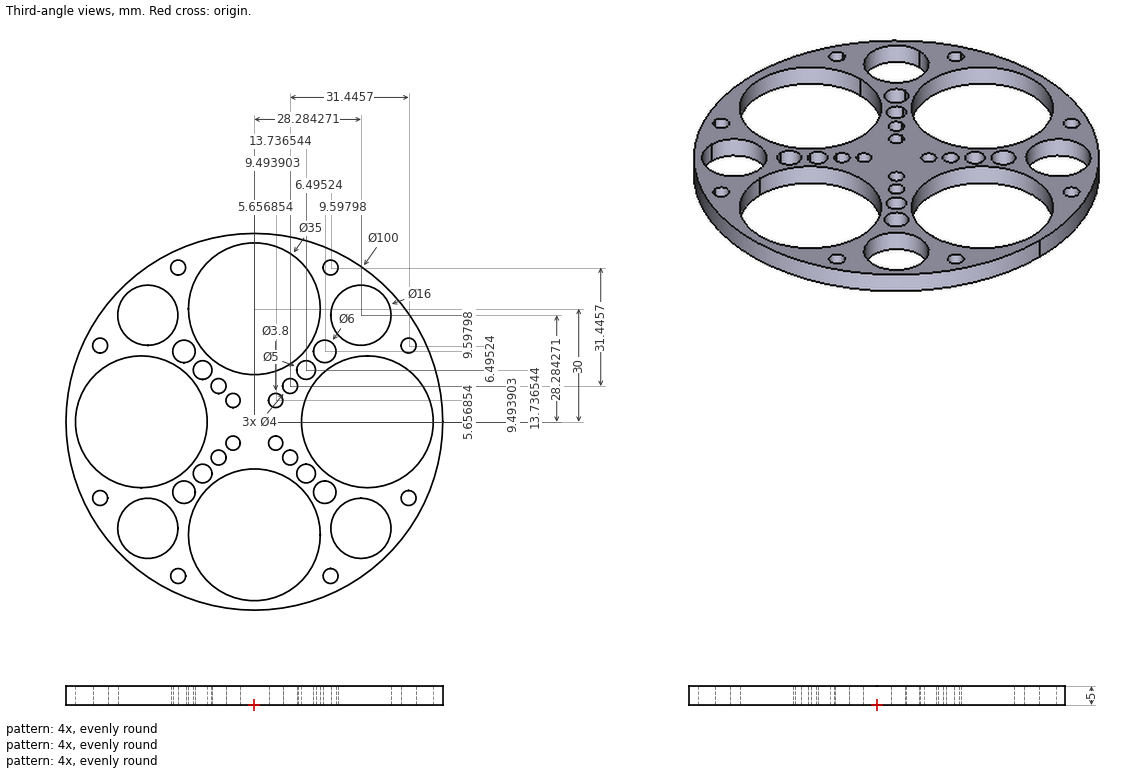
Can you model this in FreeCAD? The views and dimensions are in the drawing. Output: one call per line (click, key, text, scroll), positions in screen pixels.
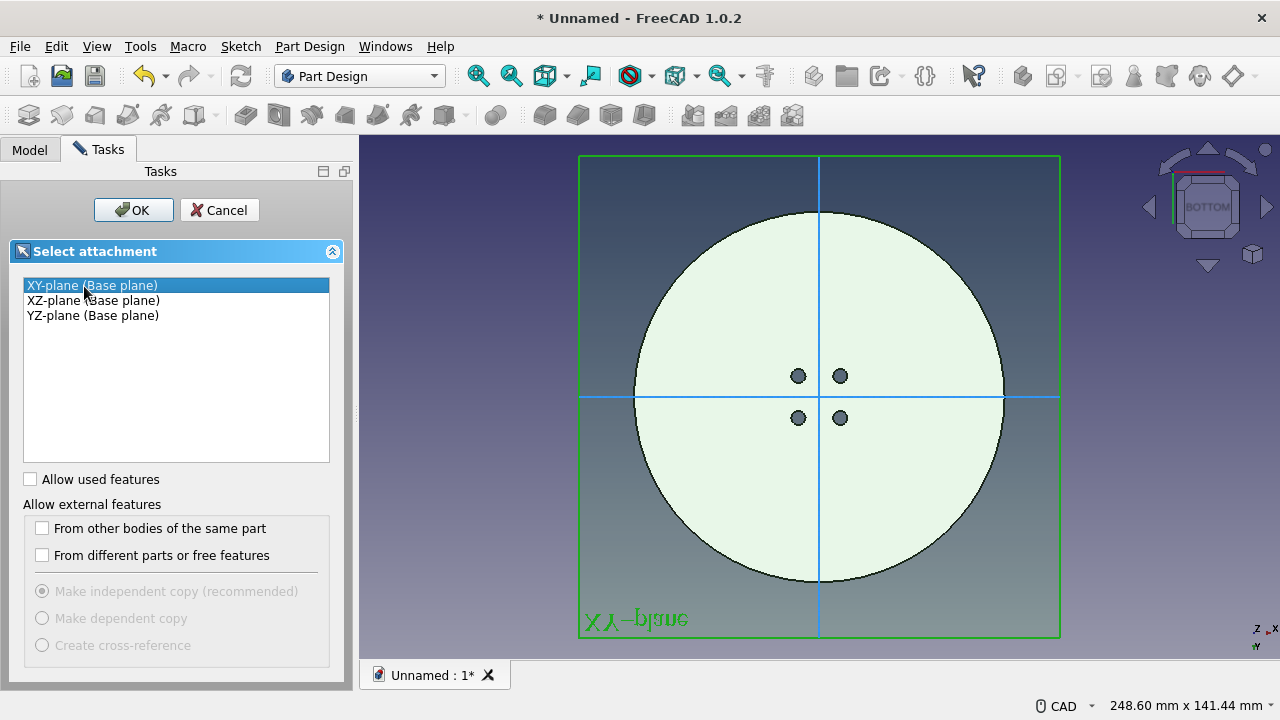
click(134, 210)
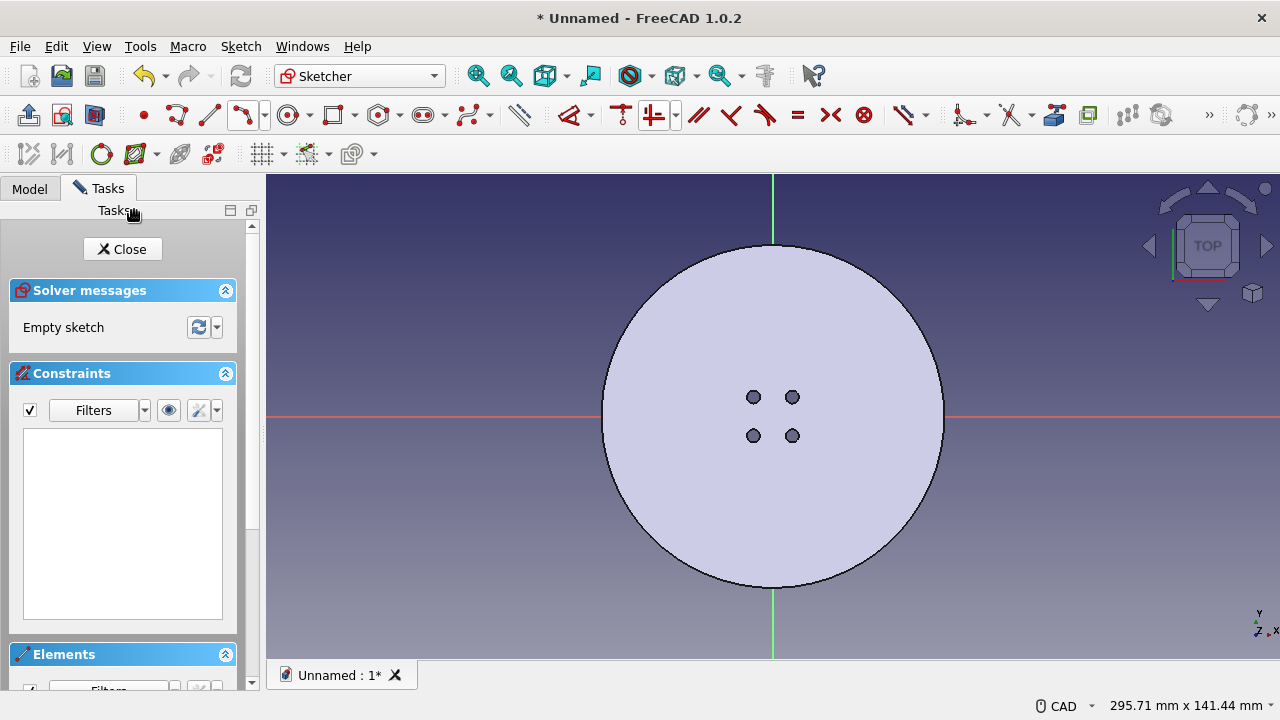
click(95, 116)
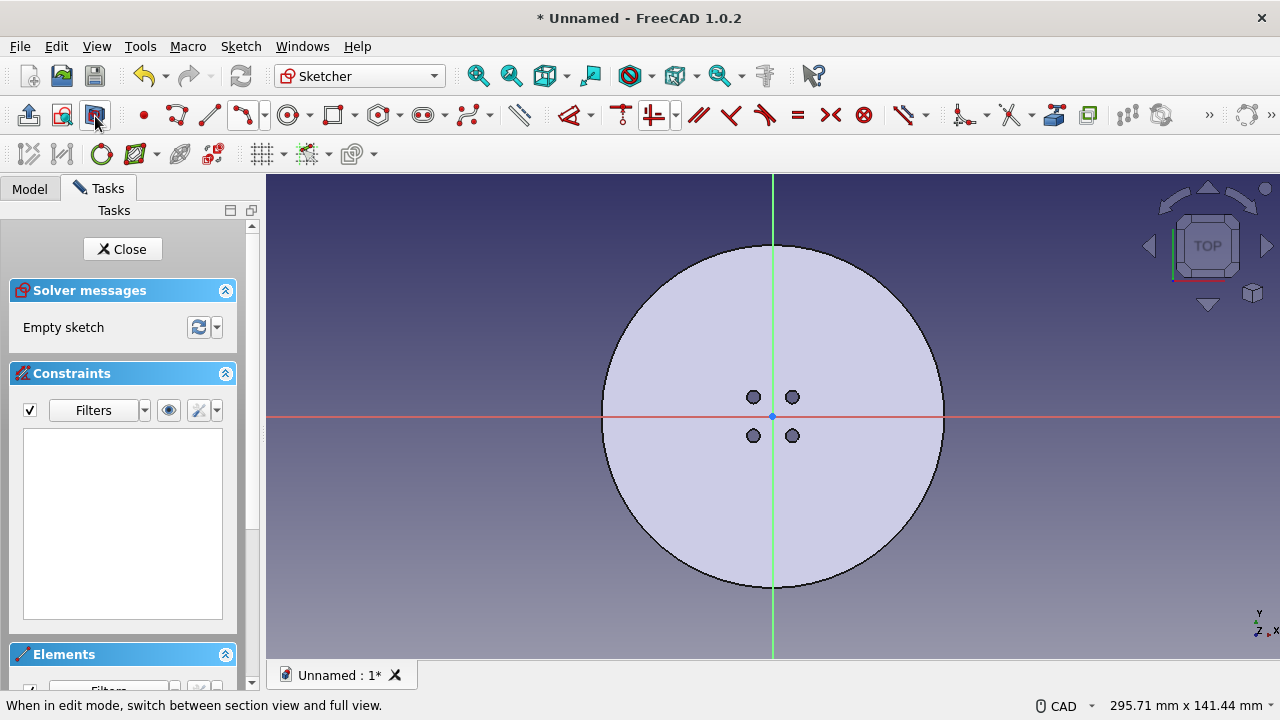
scroll(856, 236, up, 3)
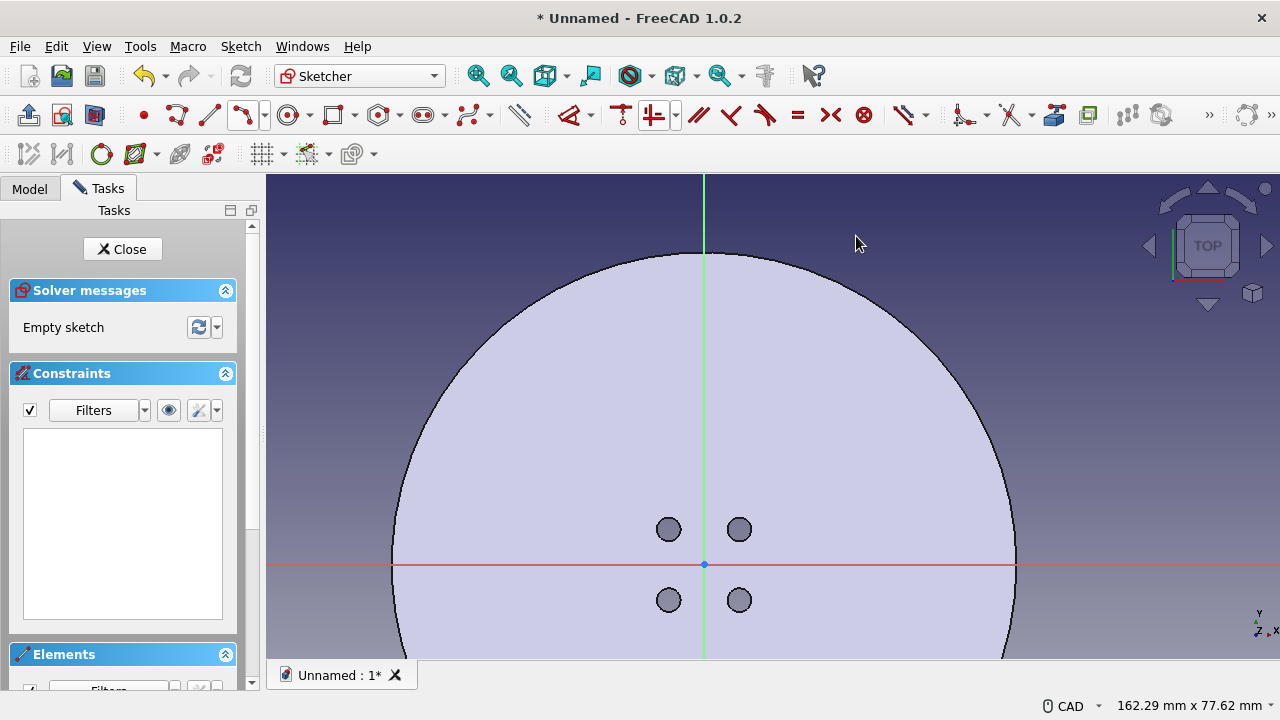
click(288, 116)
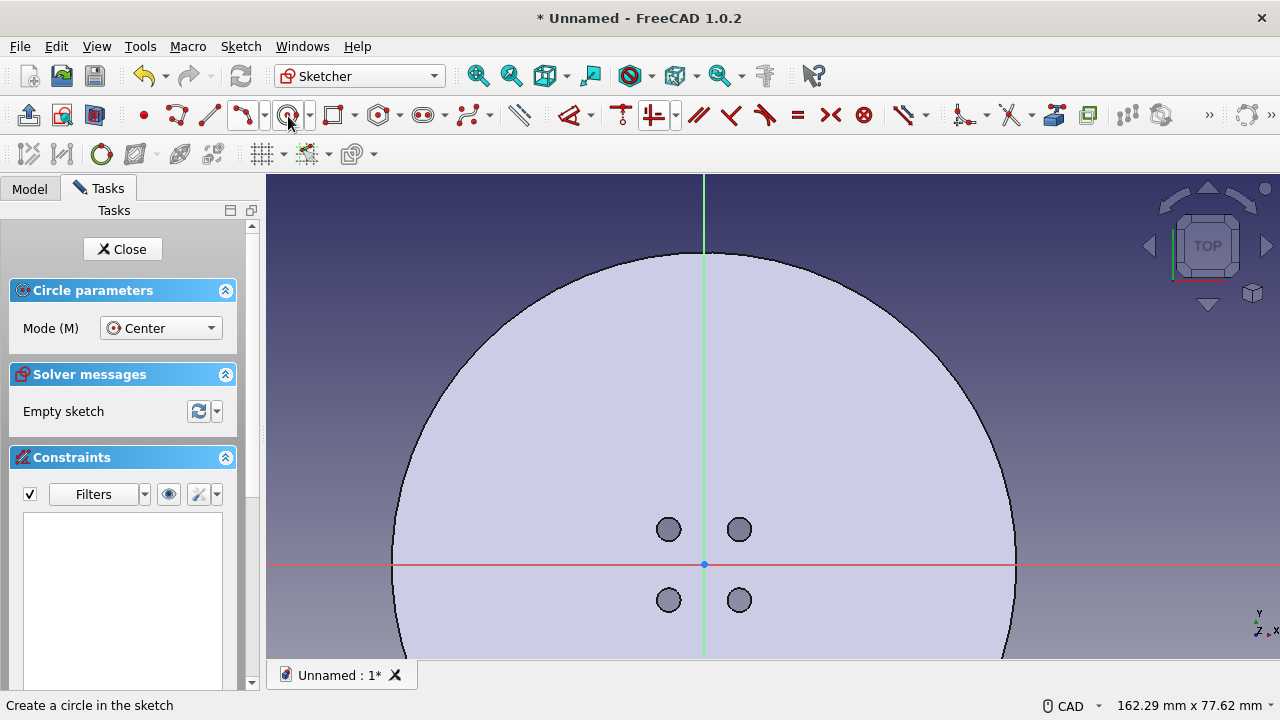
click(704, 377)
click(781, 300)
key(Escape)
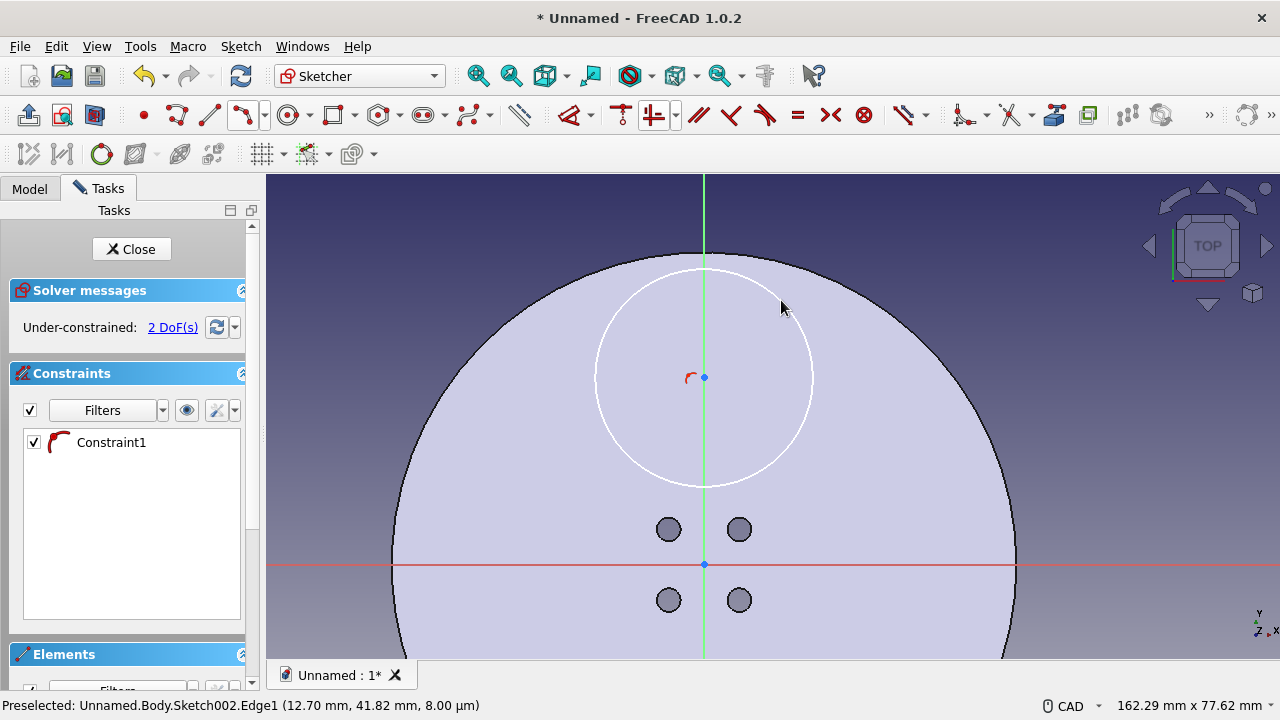
key(d)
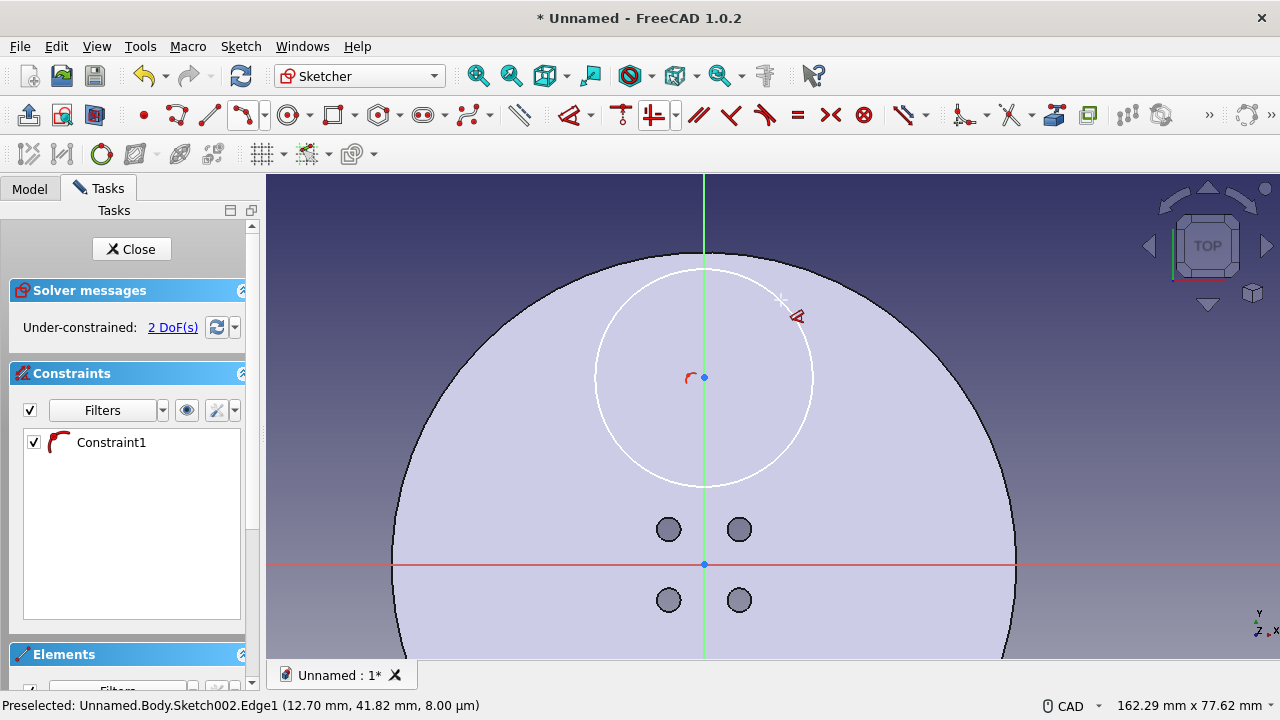
click(781, 301)
click(804, 278)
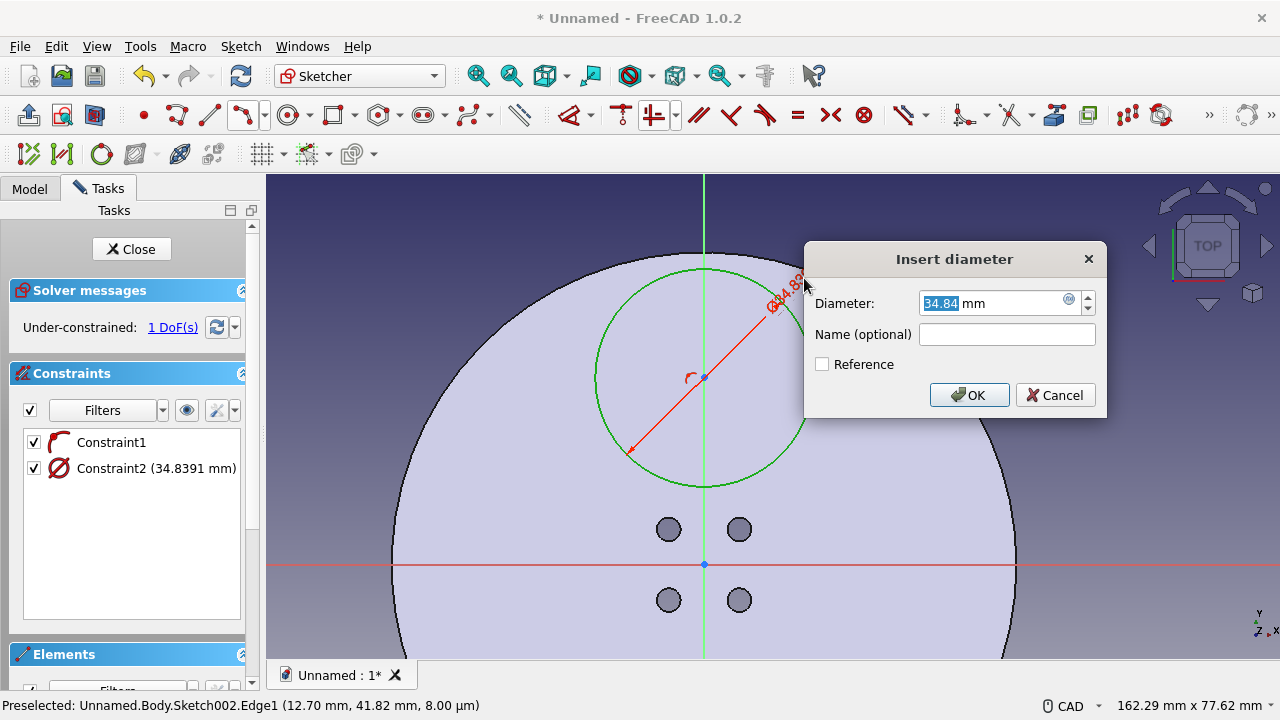
text(35)
key(Return)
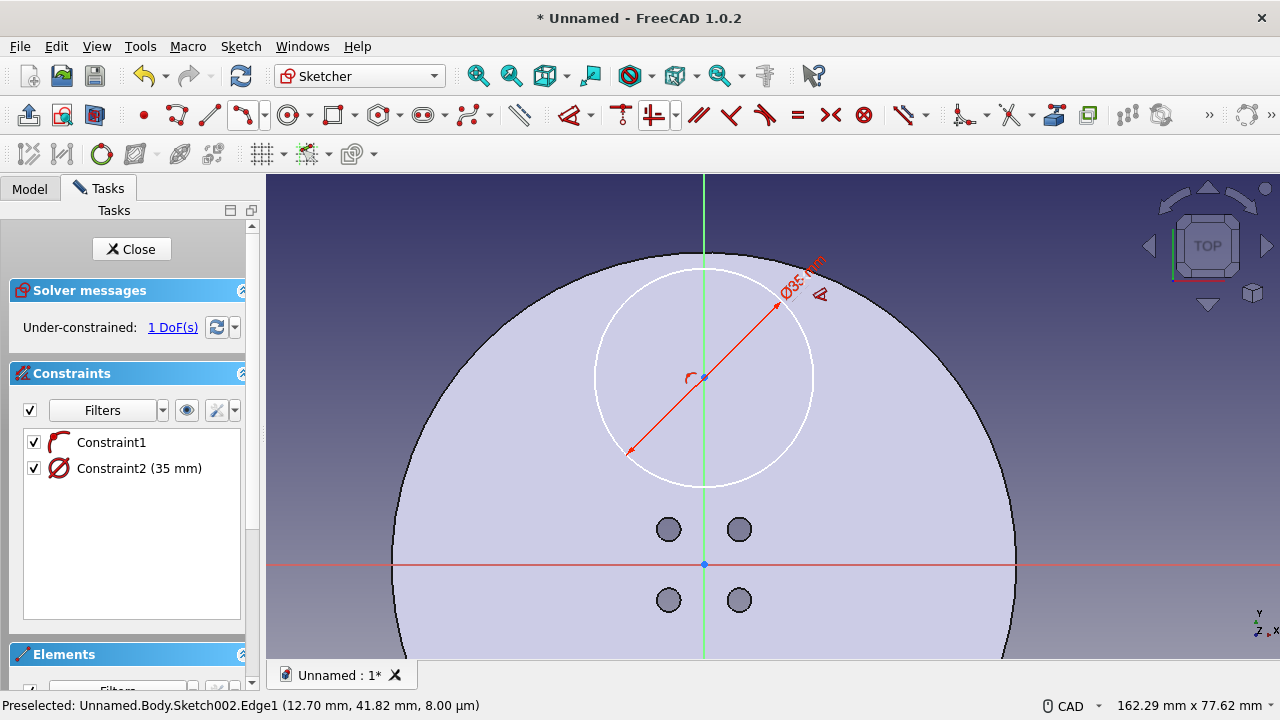
click(704, 378)
click(738, 428)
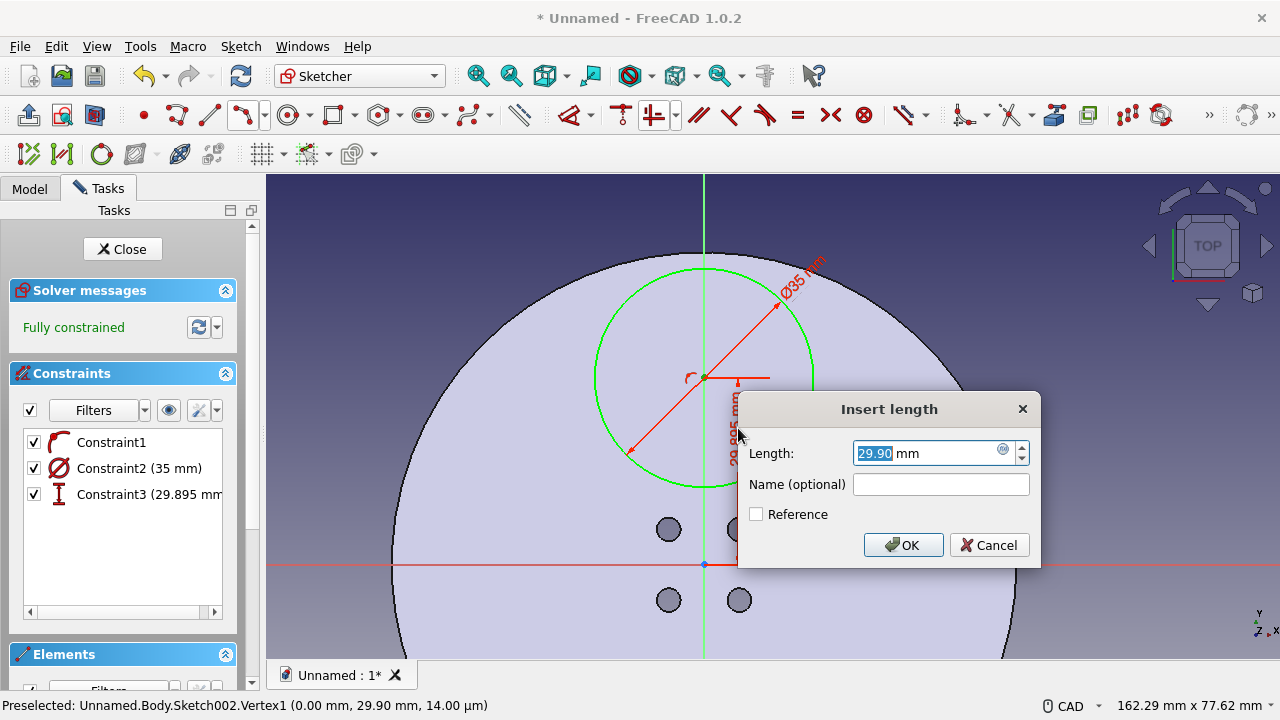
text(30)
key(Return)
key(Escape)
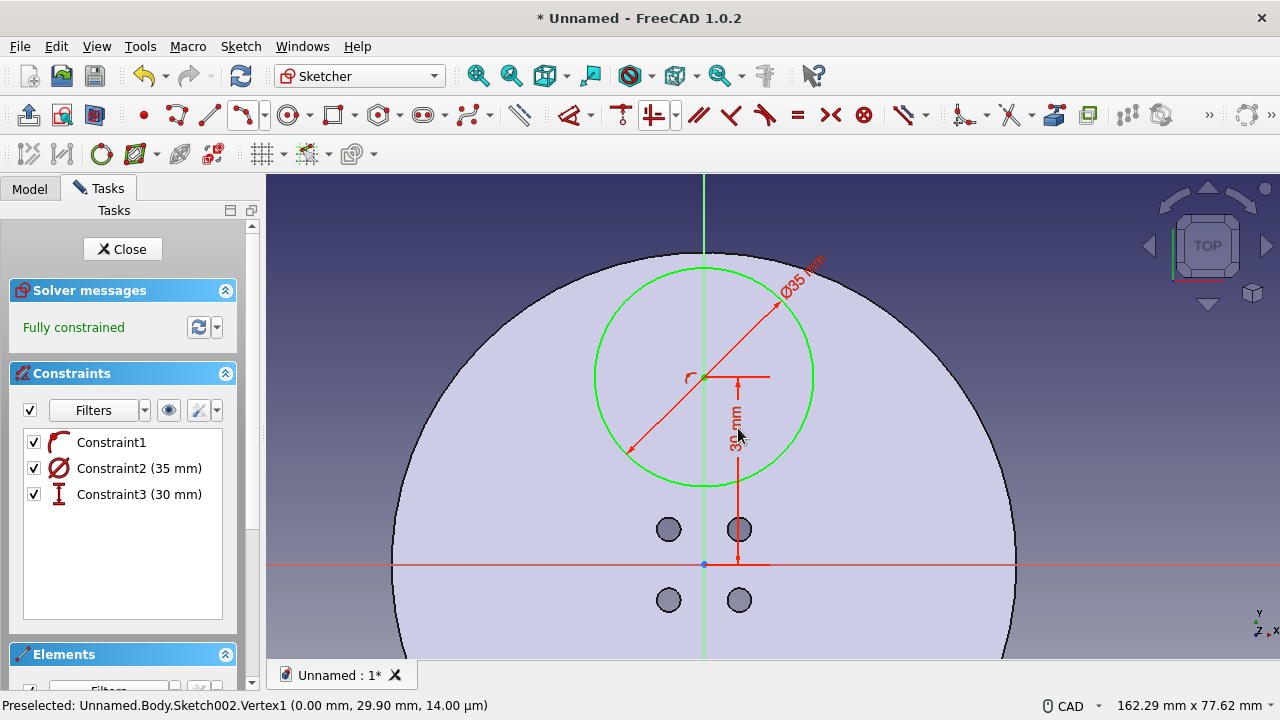
click(123, 249)